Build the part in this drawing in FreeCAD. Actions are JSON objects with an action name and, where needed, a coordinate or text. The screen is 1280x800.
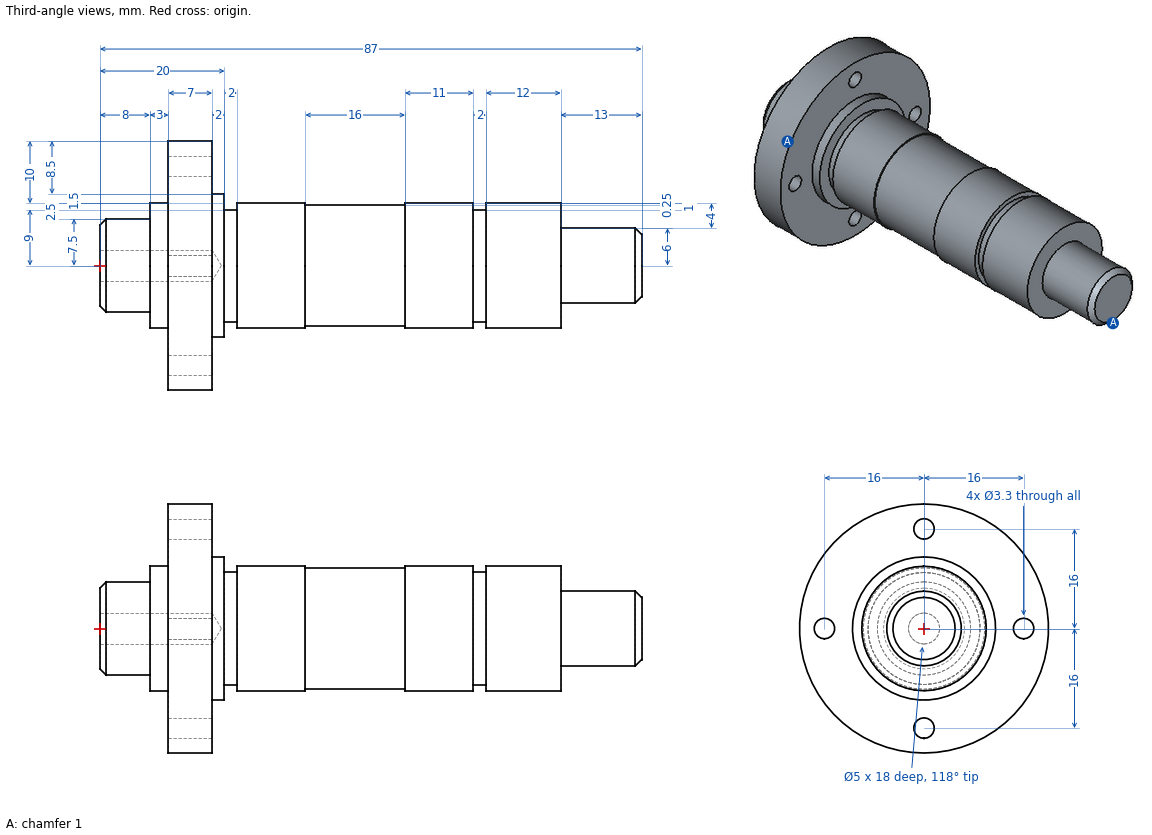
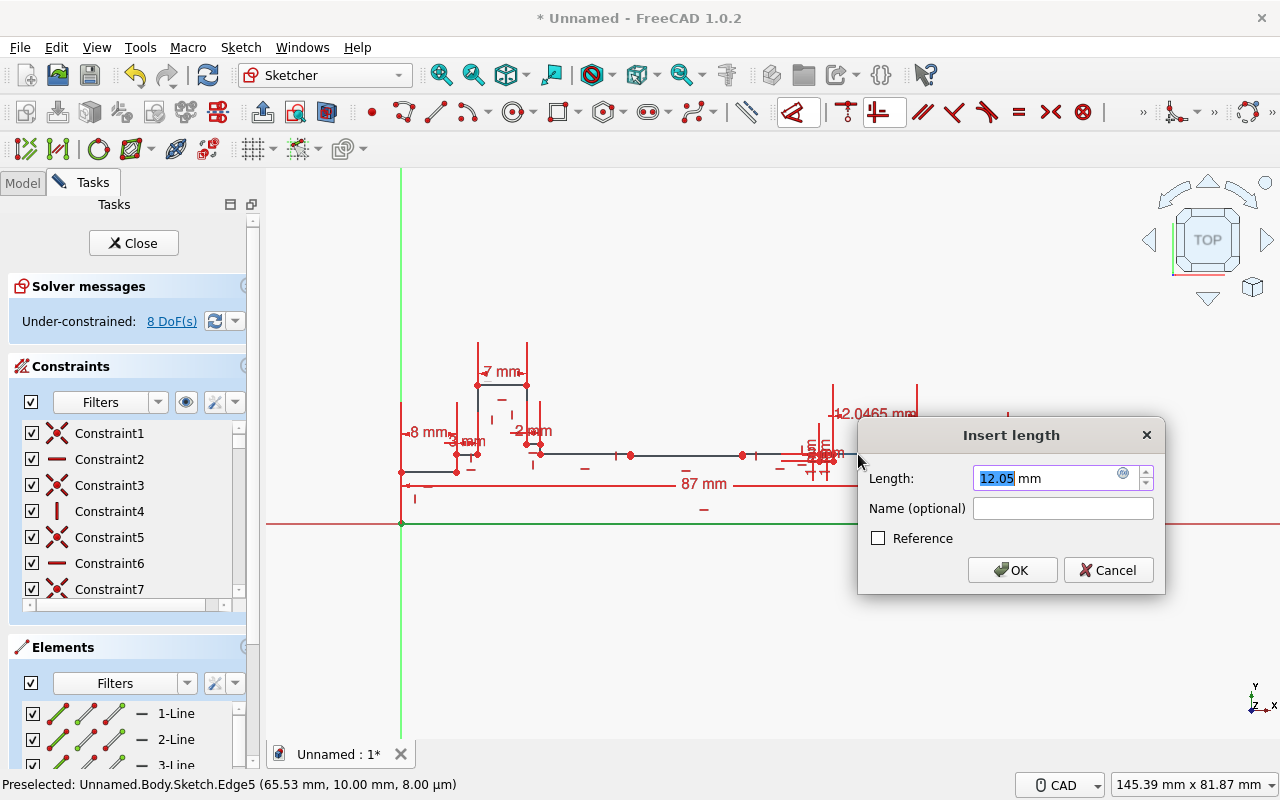
{"action": "type", "text": "12"}
{"action": "key", "text": "Return"}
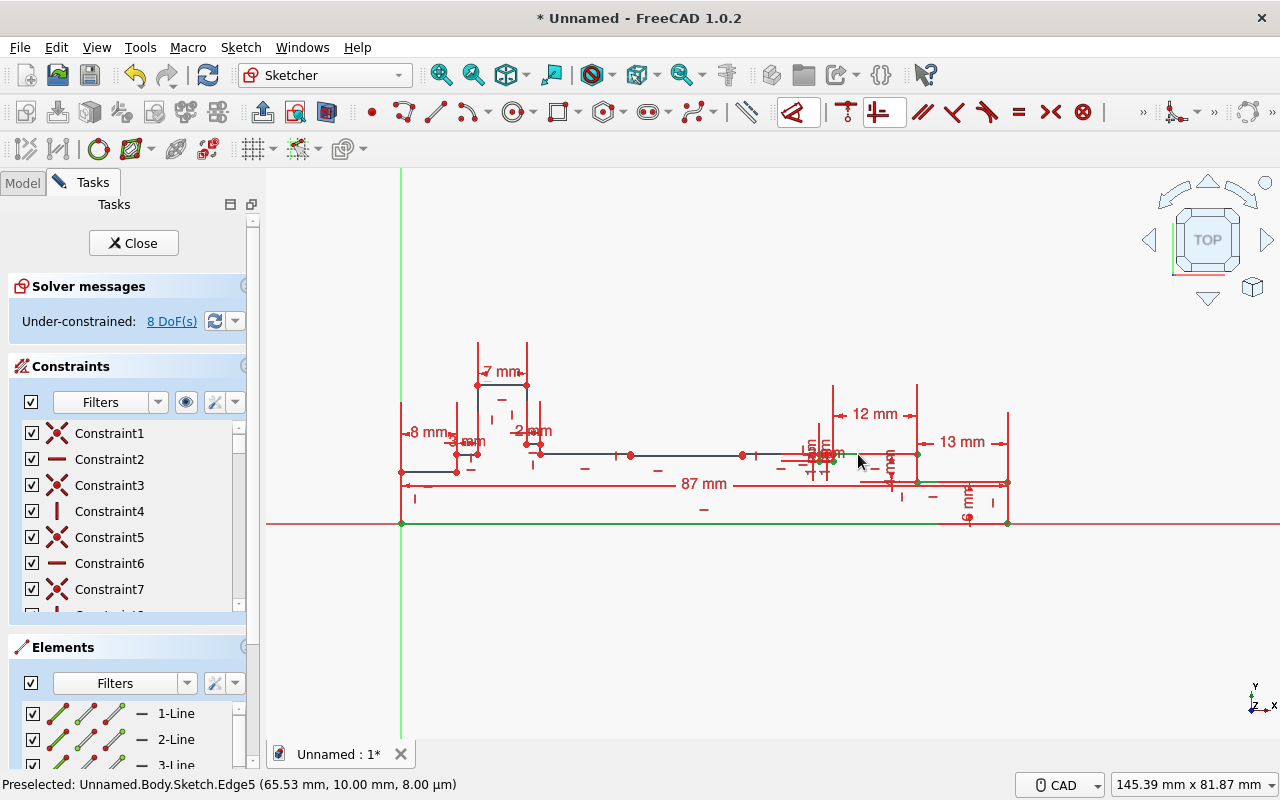
{"action": "left_click", "coordinate": [796, 454]}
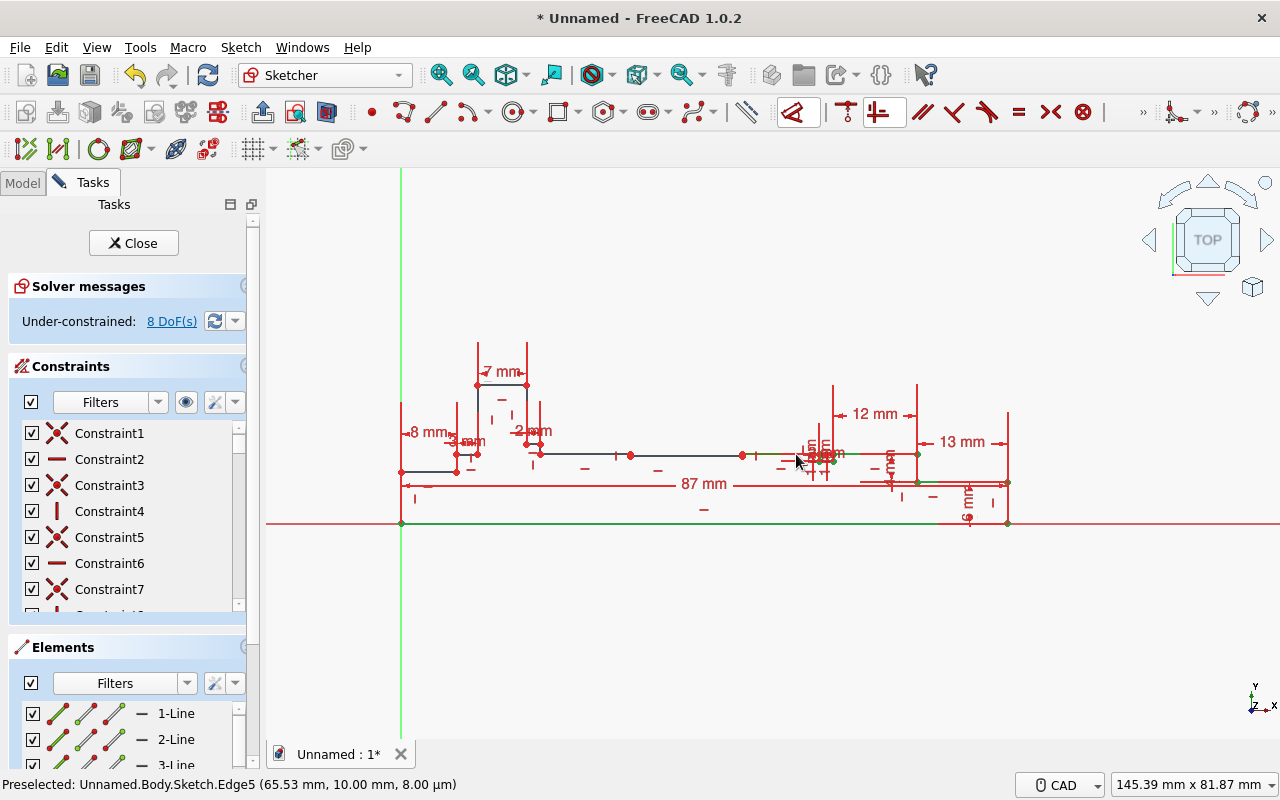
{"action": "left_click", "coordinate": [814, 112]}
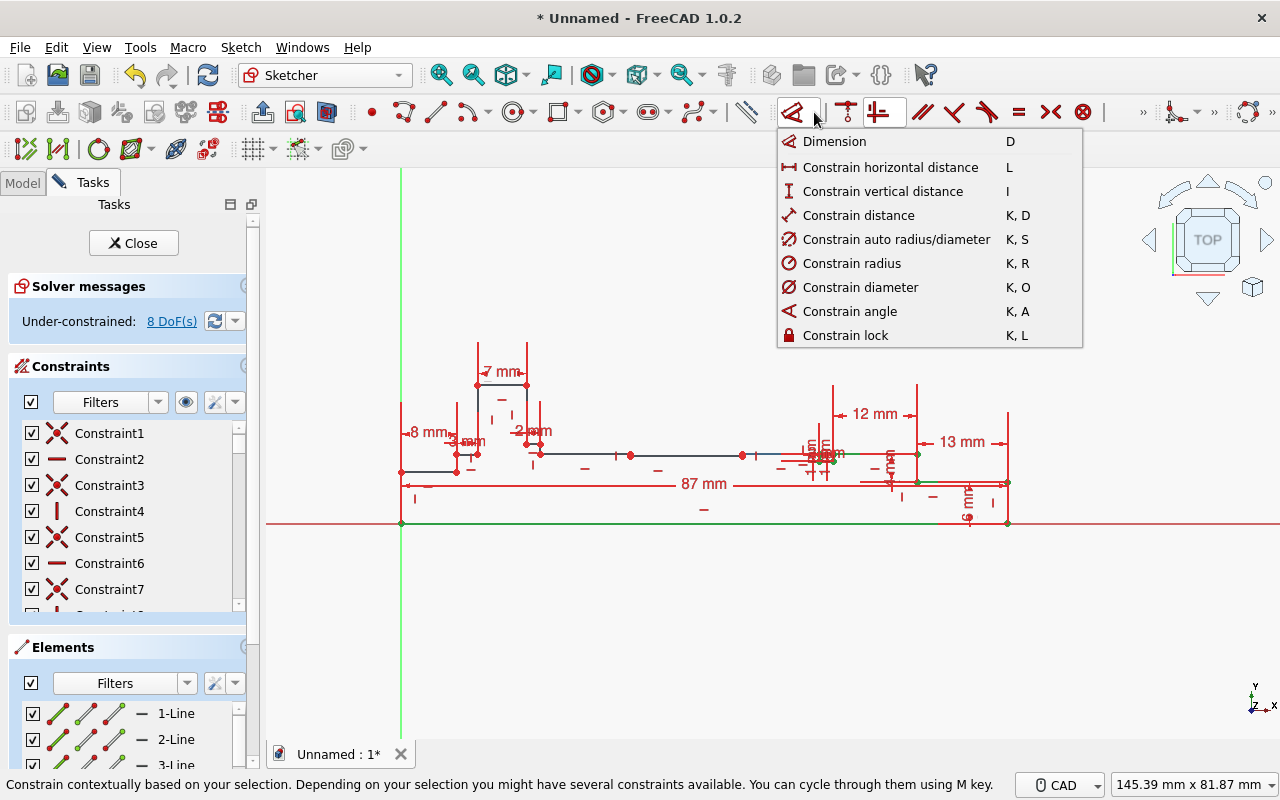
{"action": "left_click", "coordinate": [930, 167]}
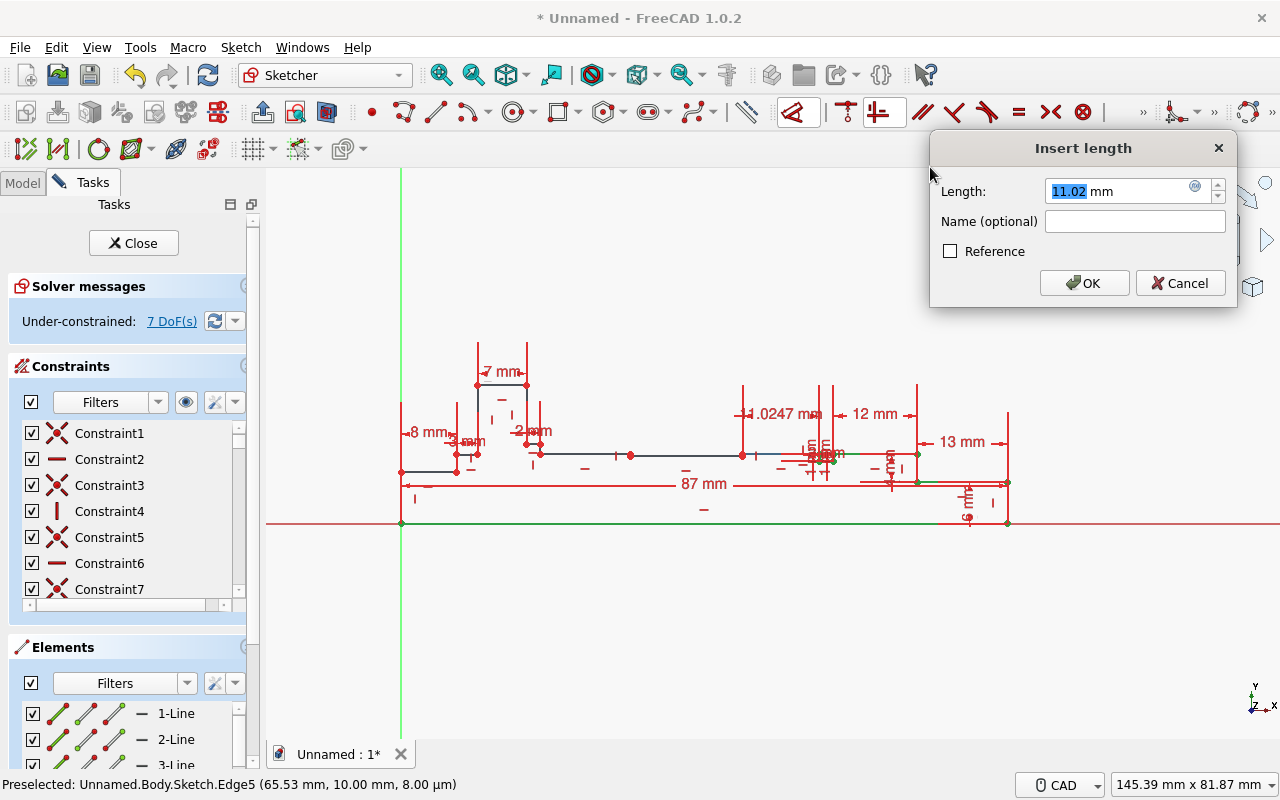
{"action": "type", "text": "11"}
{"action": "key", "text": "Return"}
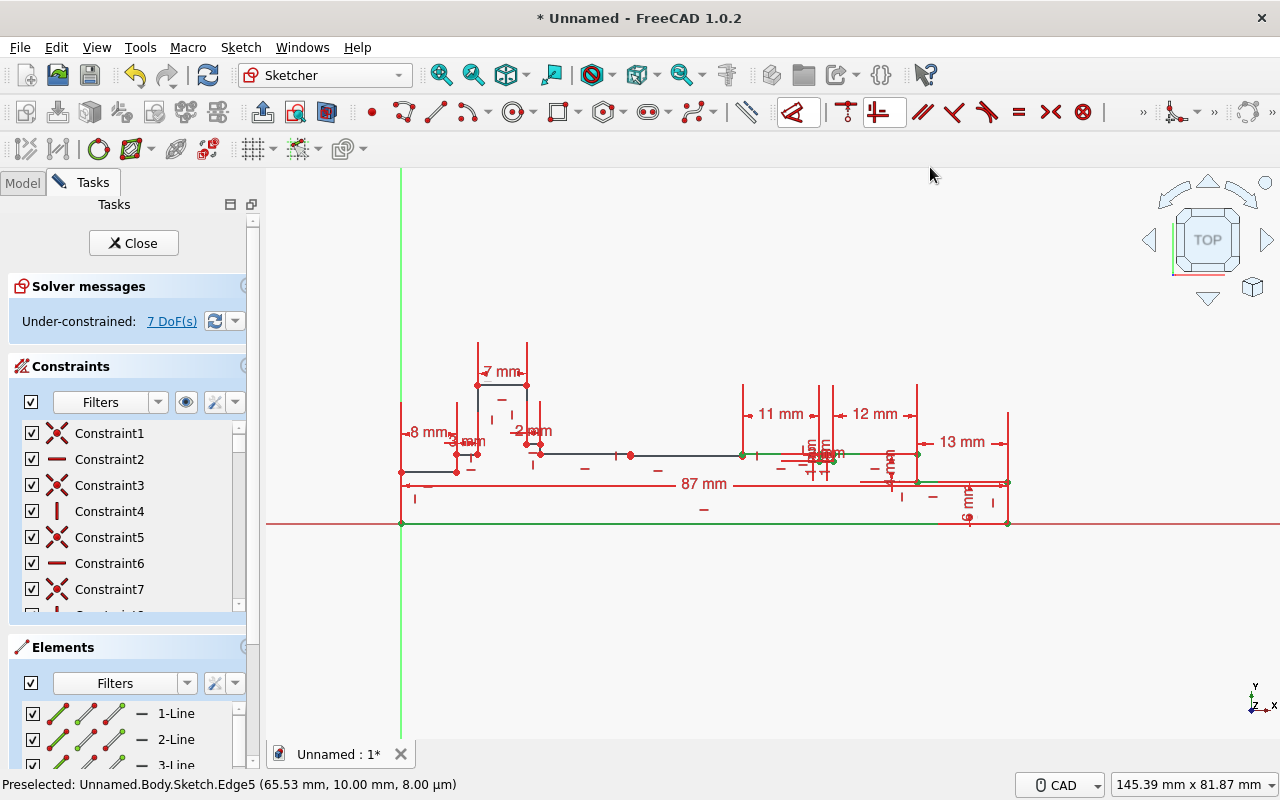
{"action": "left_click", "coordinate": [709, 456]}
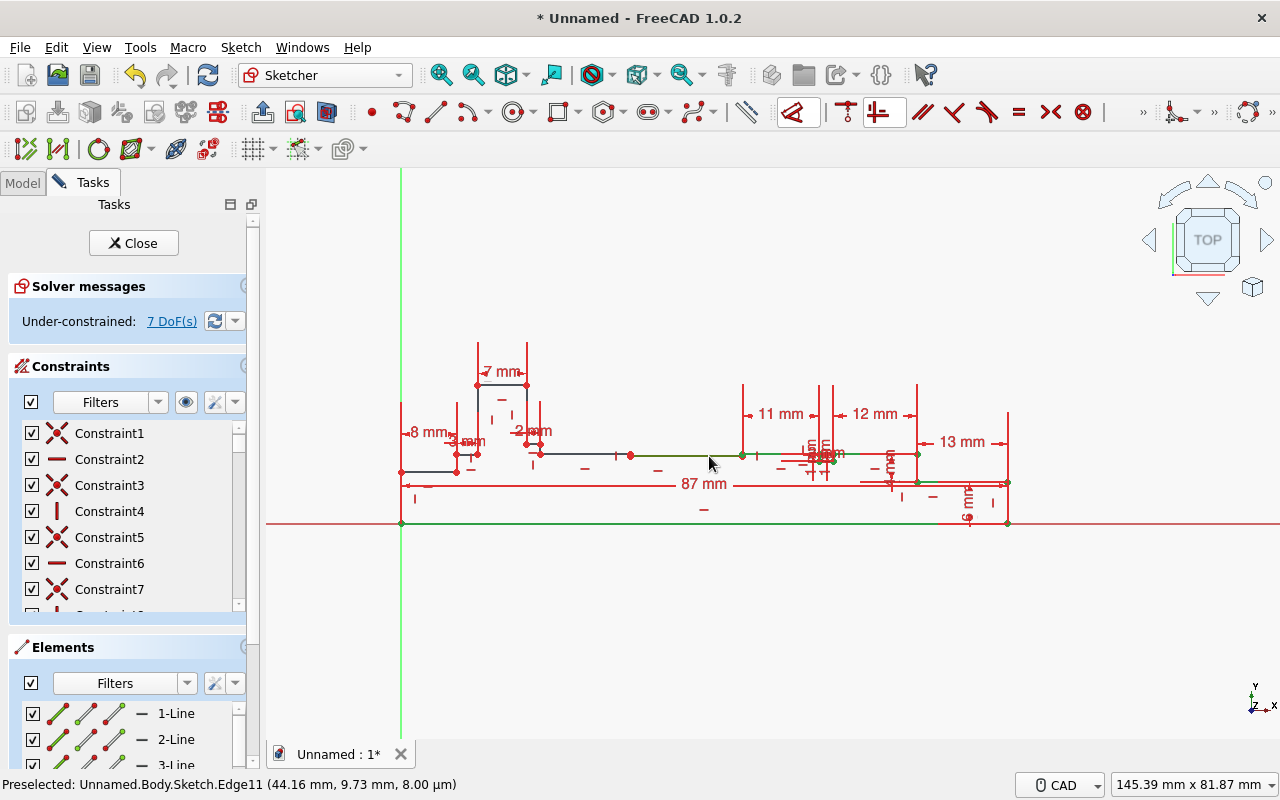
{"action": "left_click", "coordinate": [814, 112]}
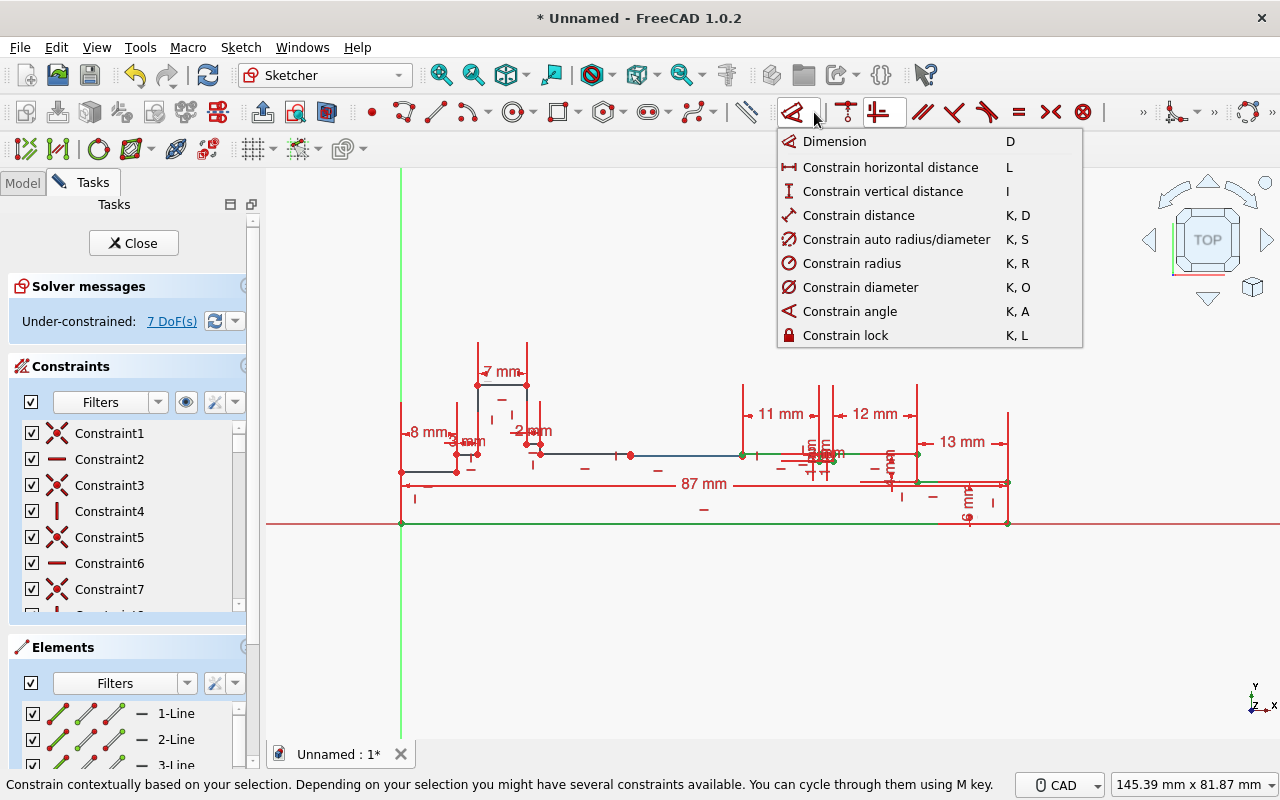
{"action": "left_click", "coordinate": [930, 167]}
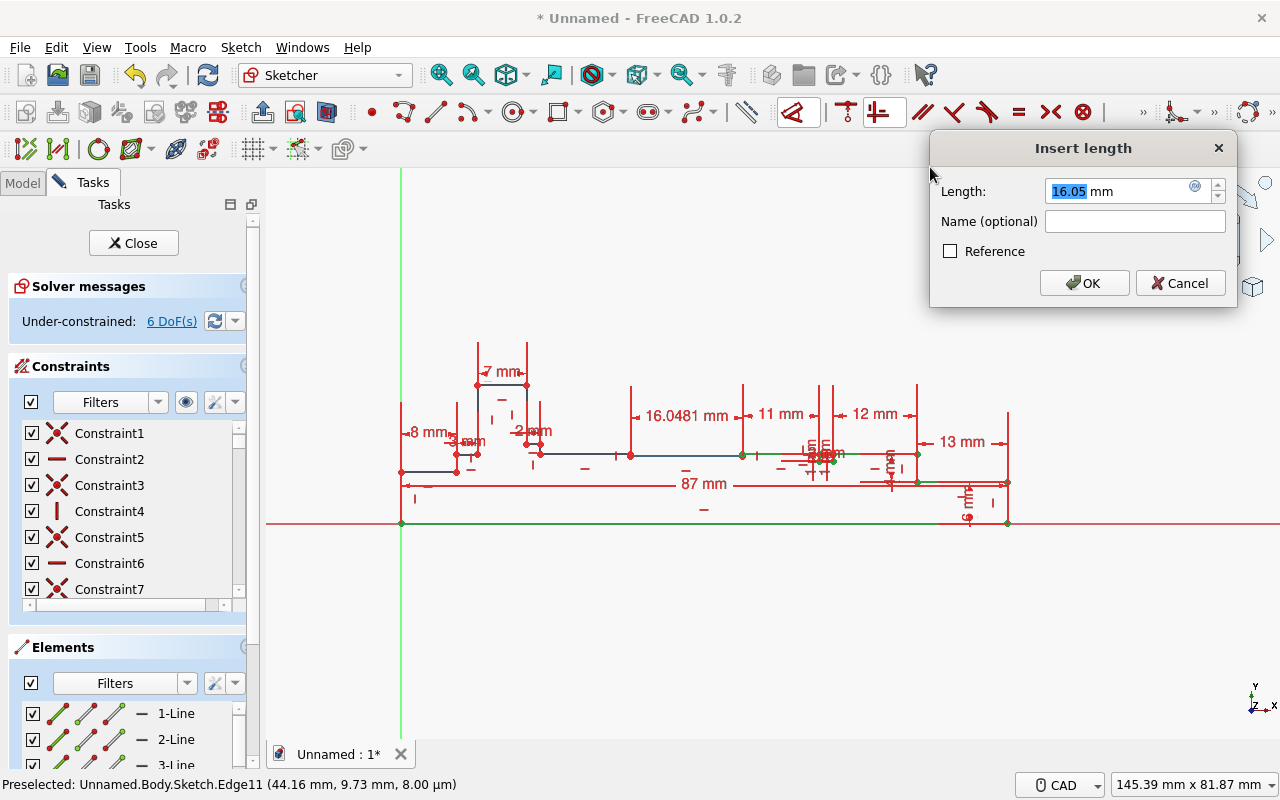
{"action": "type", "text": "16"}
{"action": "key", "text": "Return"}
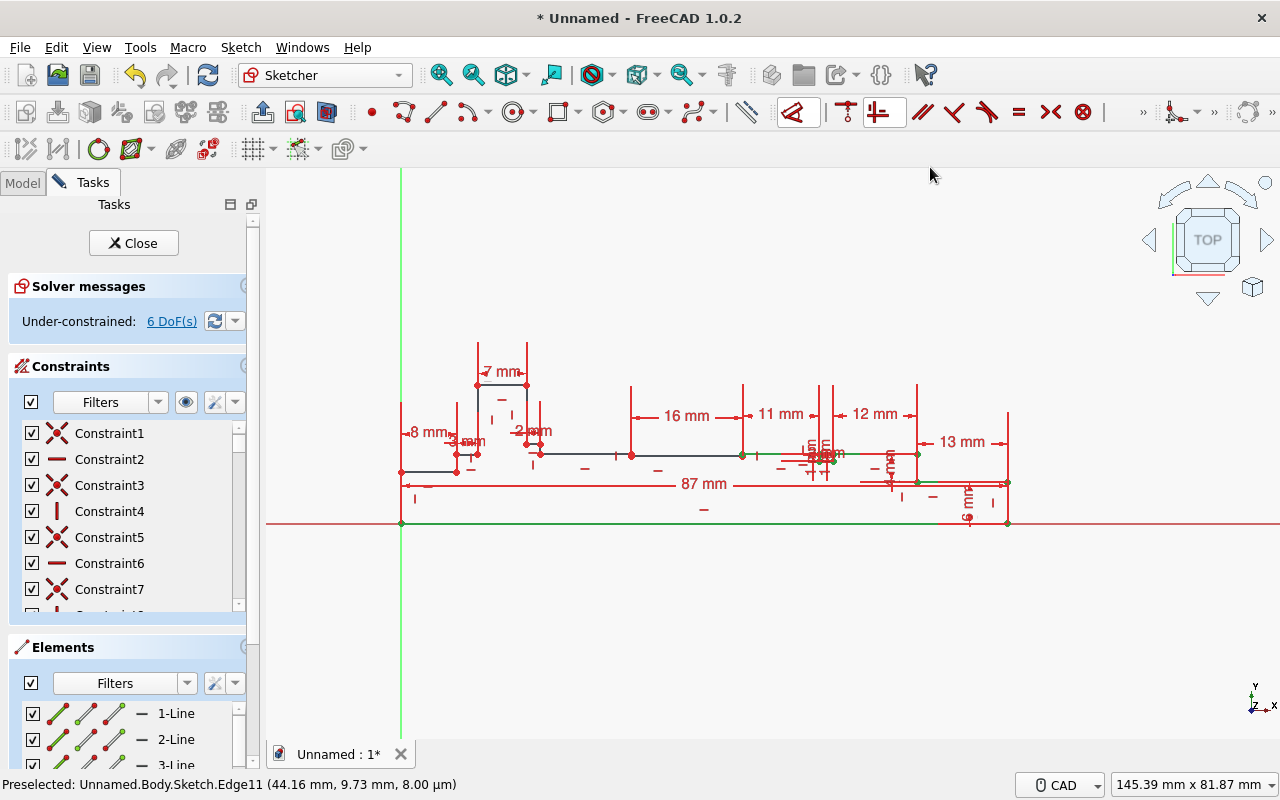
{"action": "left_click", "coordinate": [478, 406]}